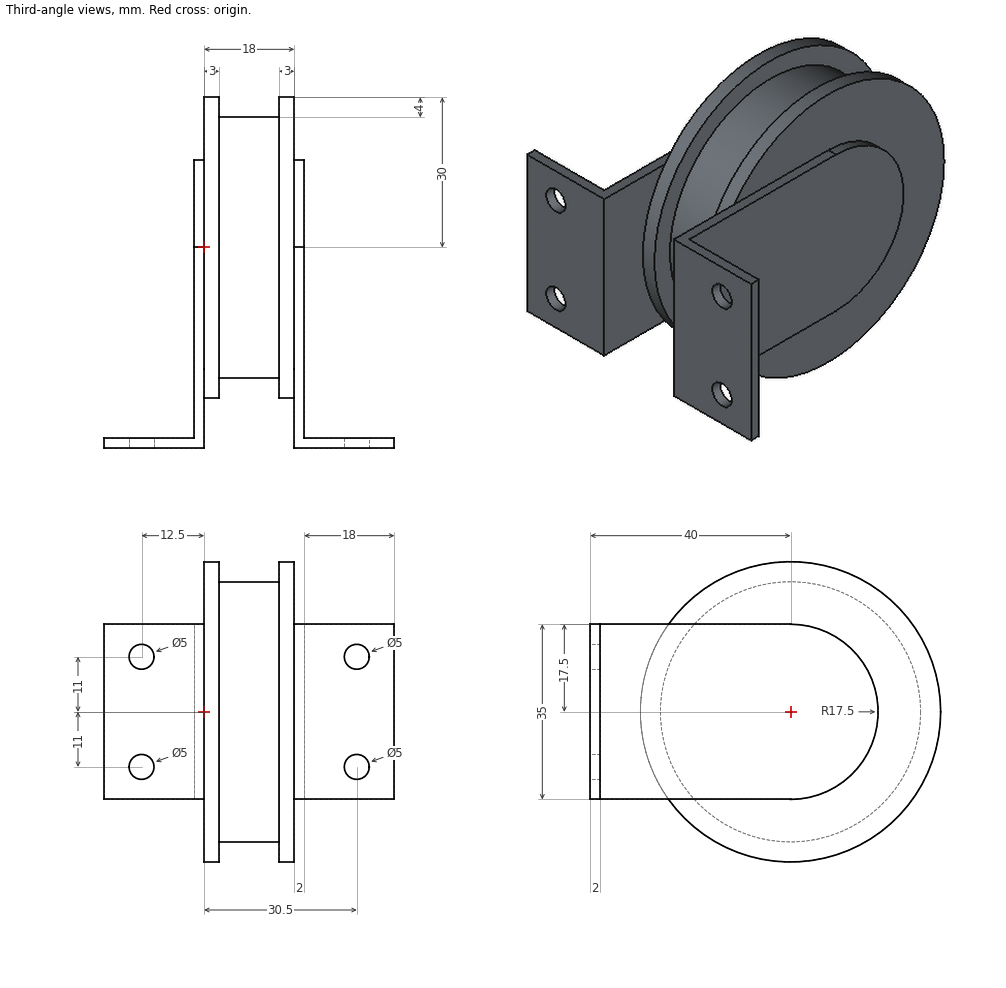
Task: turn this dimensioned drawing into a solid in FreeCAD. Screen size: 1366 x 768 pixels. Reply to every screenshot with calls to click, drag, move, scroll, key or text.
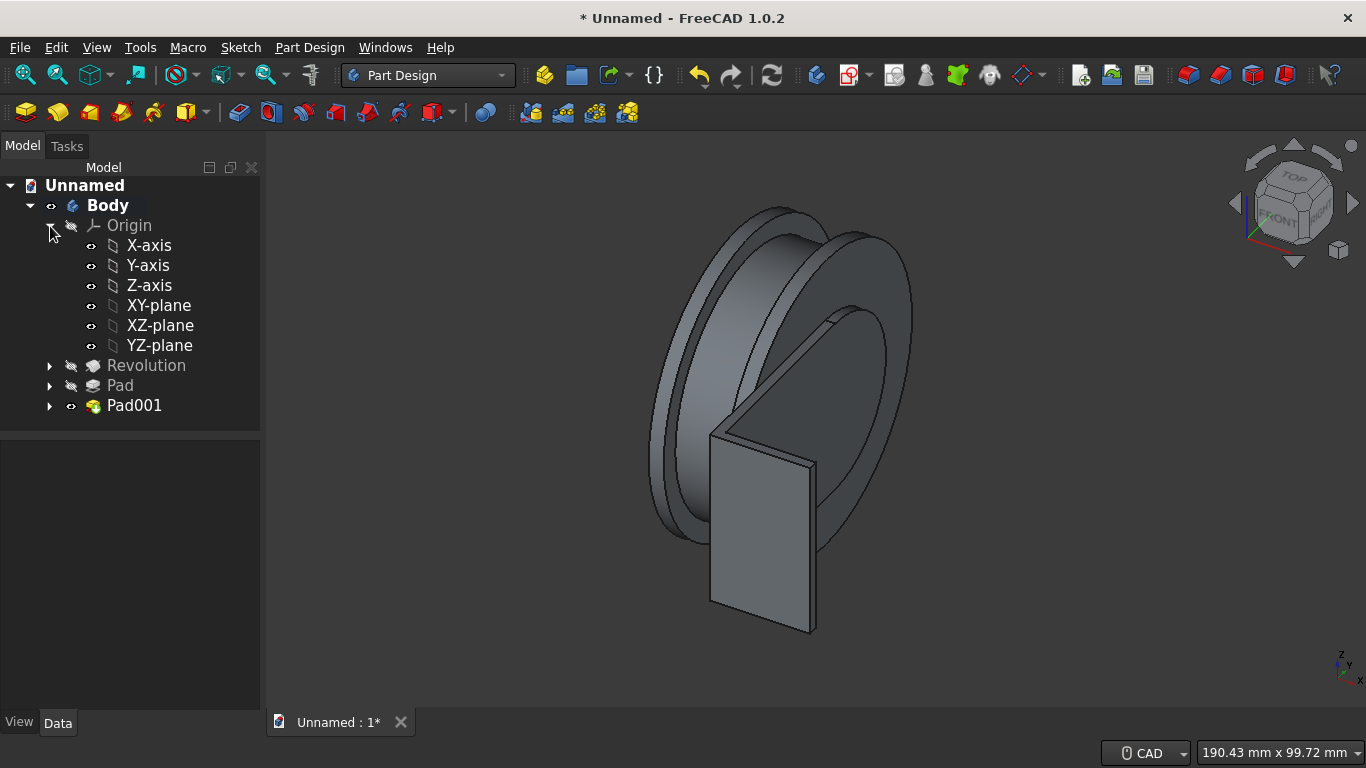
click(136, 346)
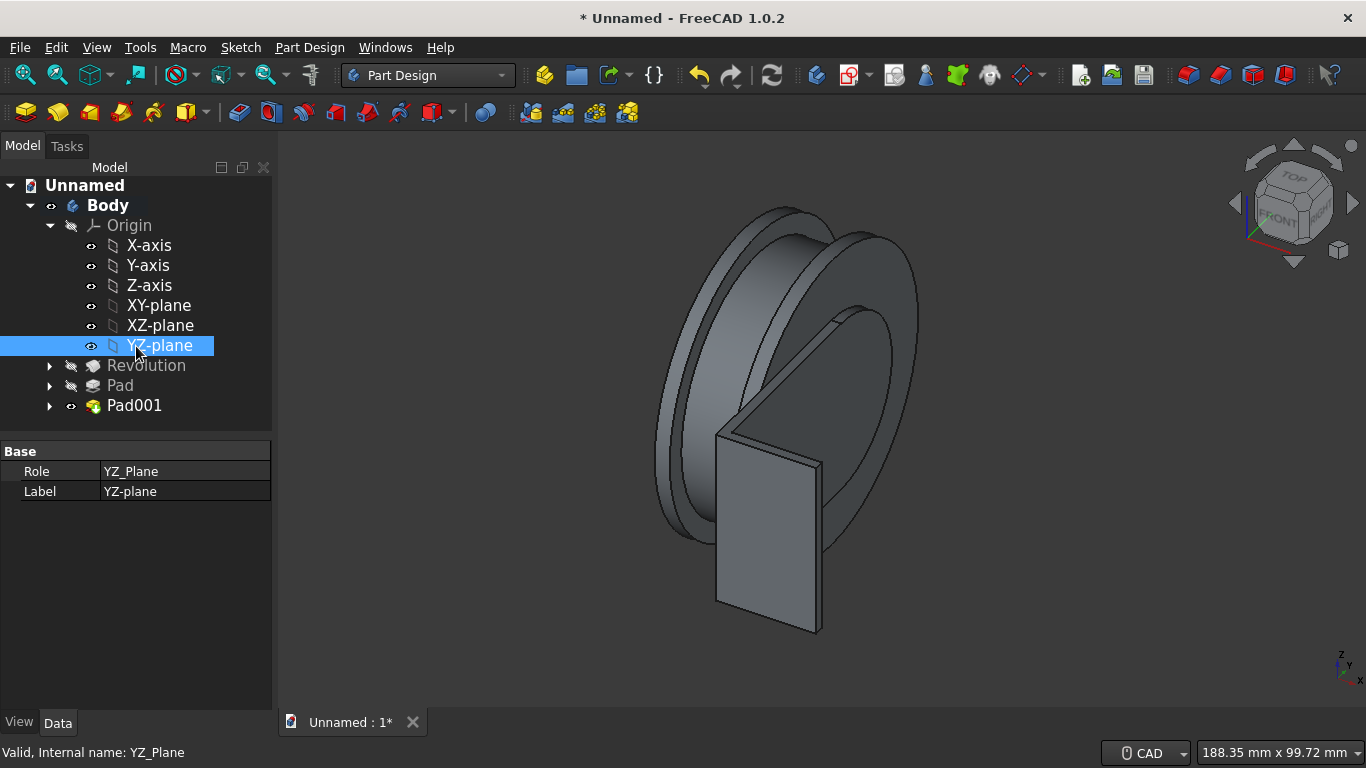
click(1022, 76)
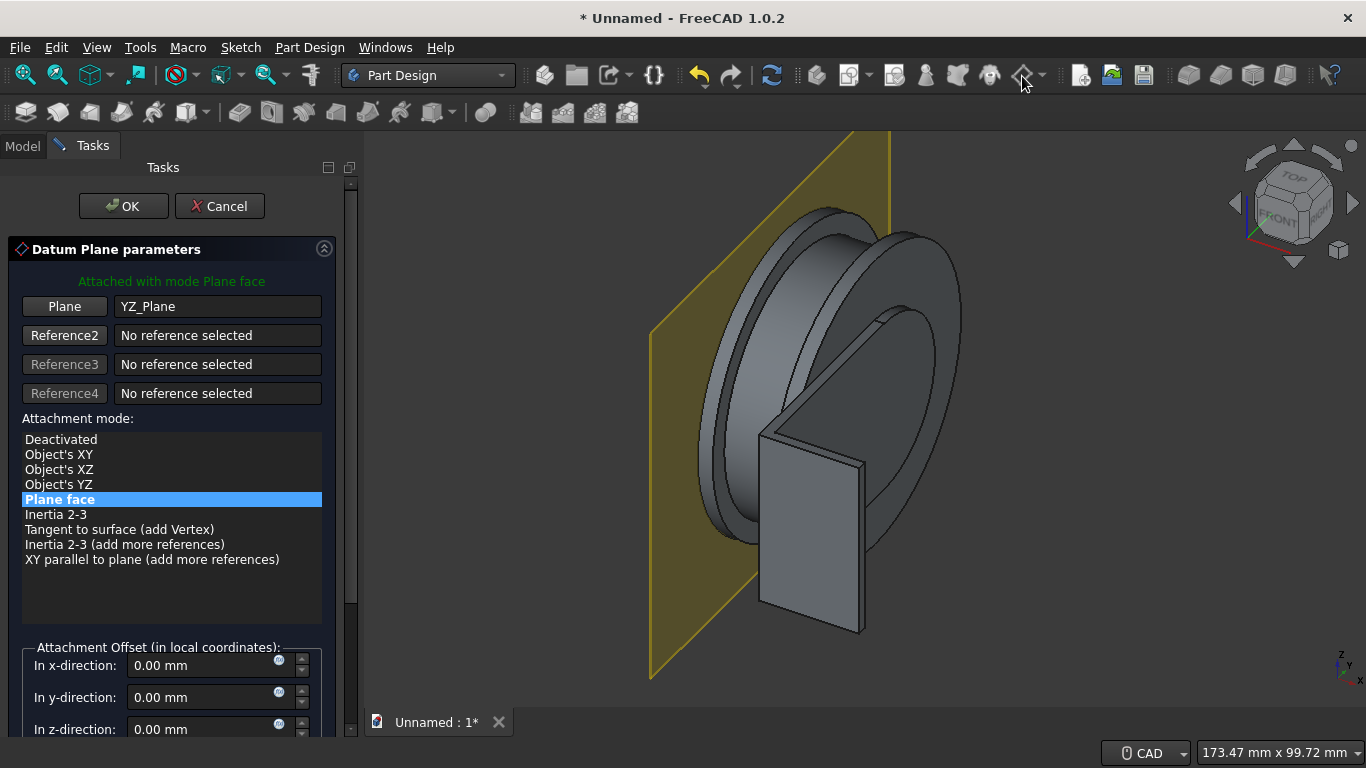
scroll(351, 456, down, 2)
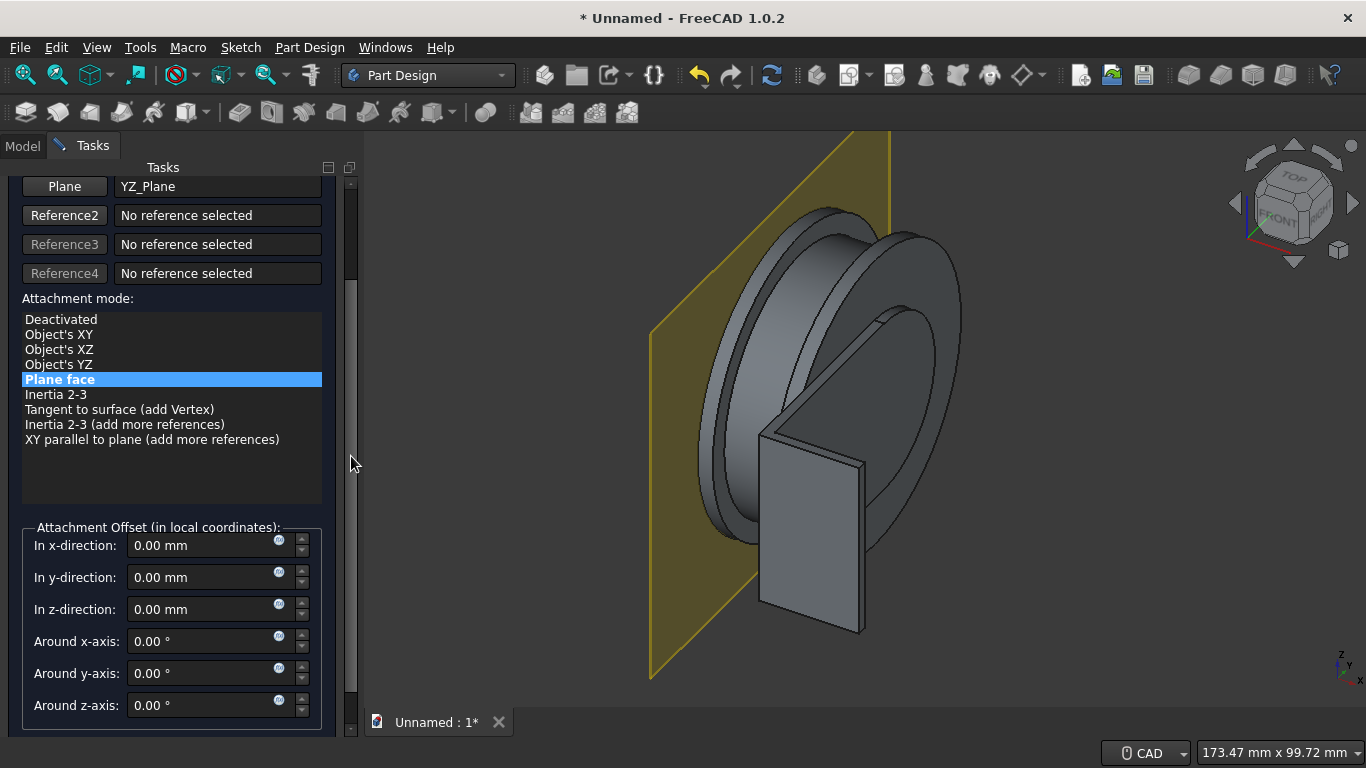
triple_click(210, 609)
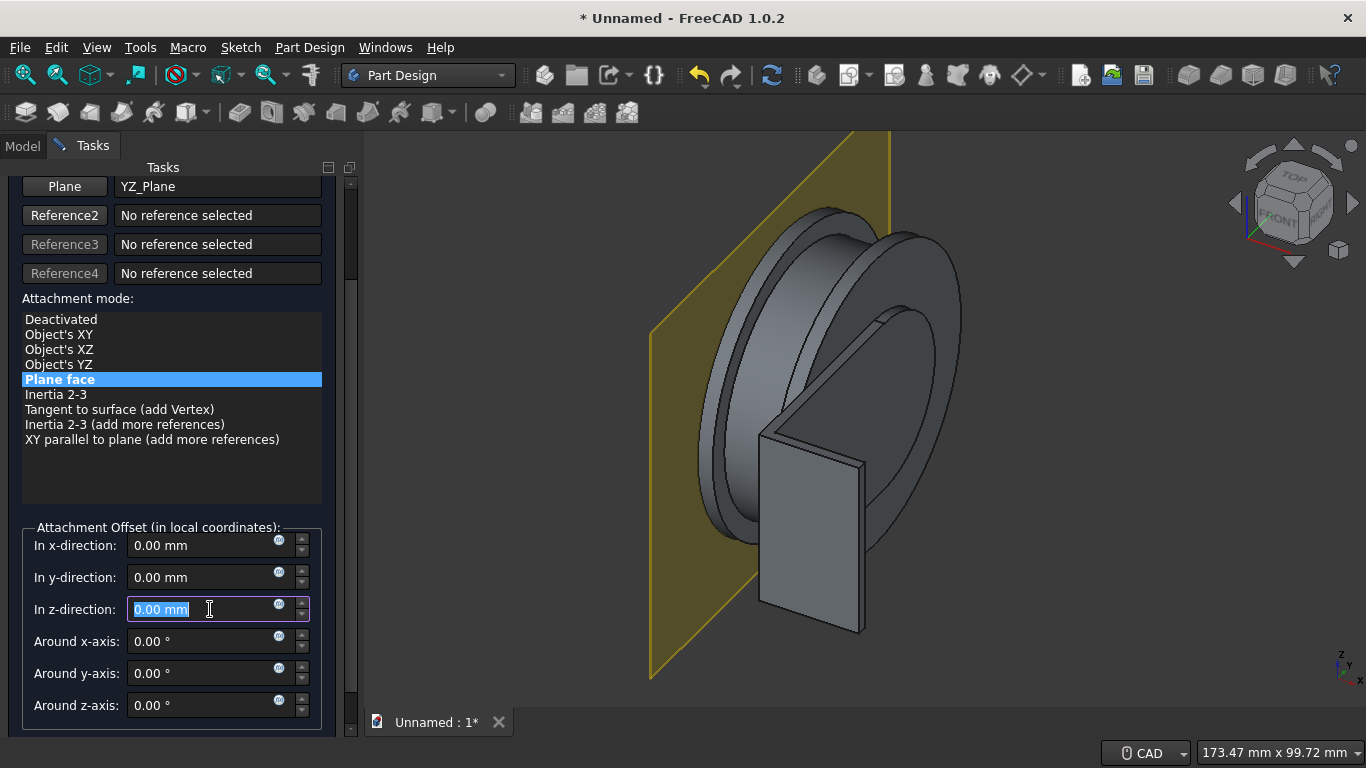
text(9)
key(Tab)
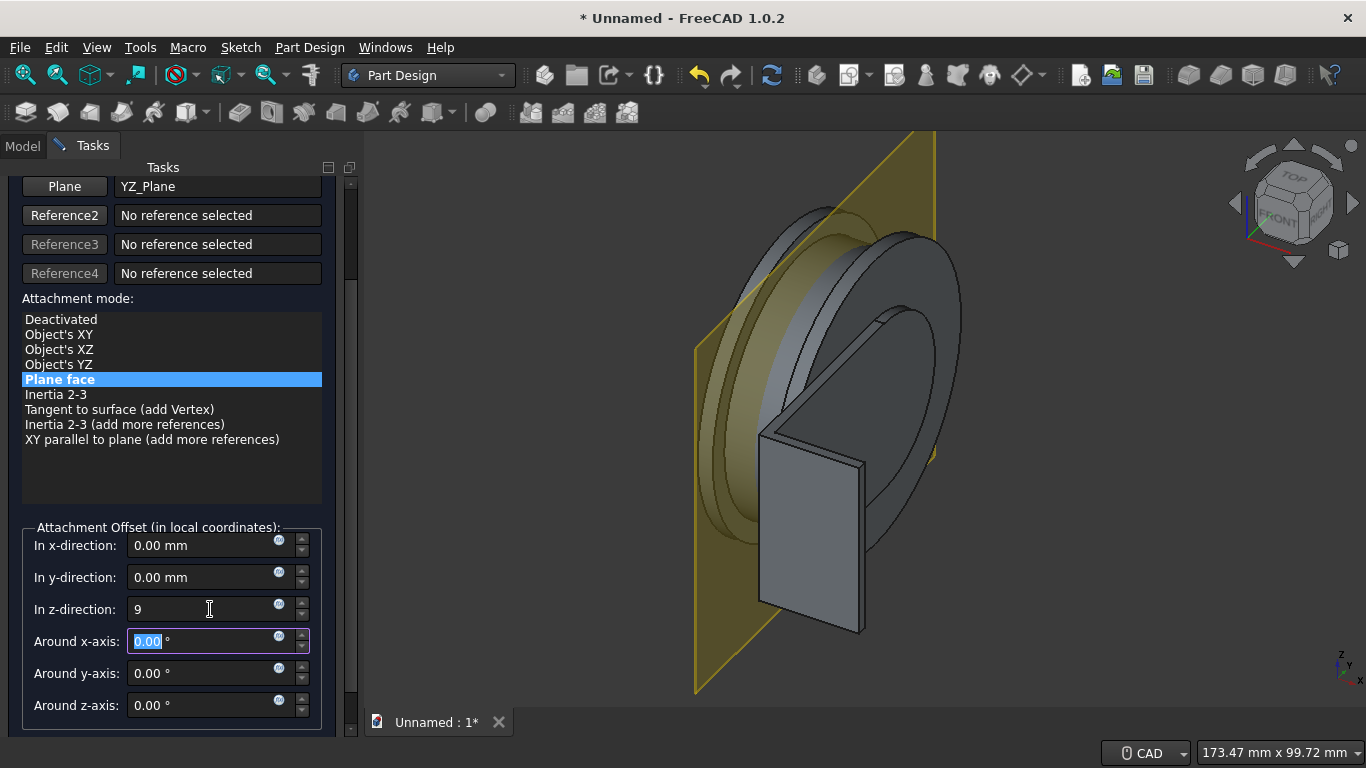
scroll(351, 456, up, 3)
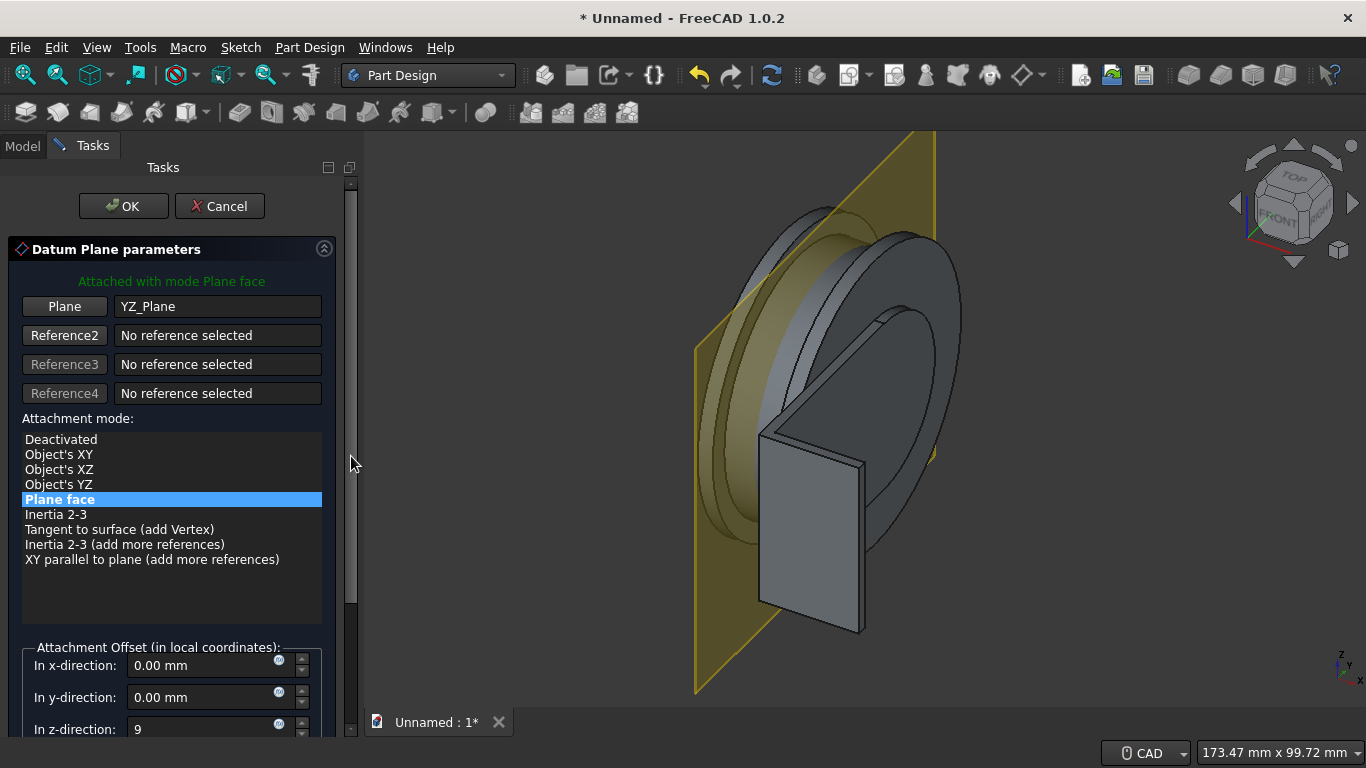
click(124, 206)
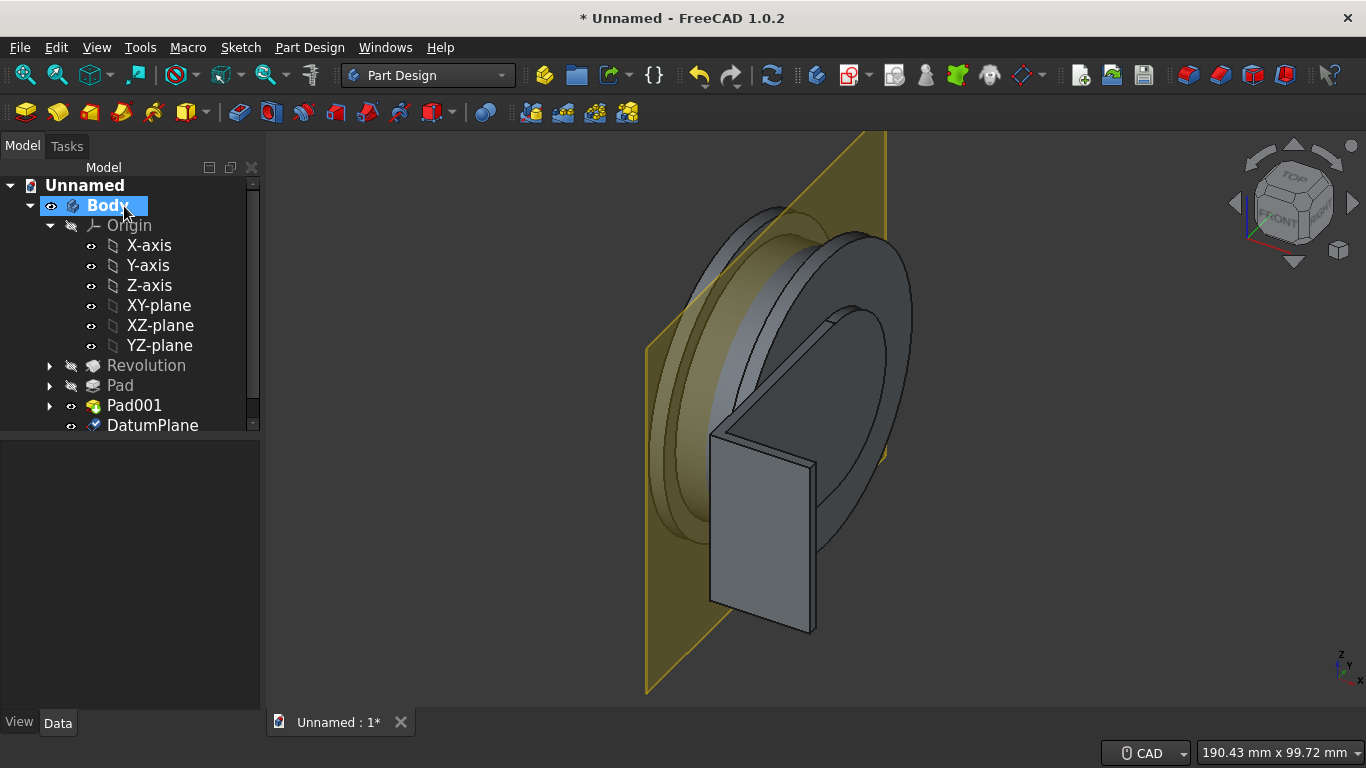
click(116, 386)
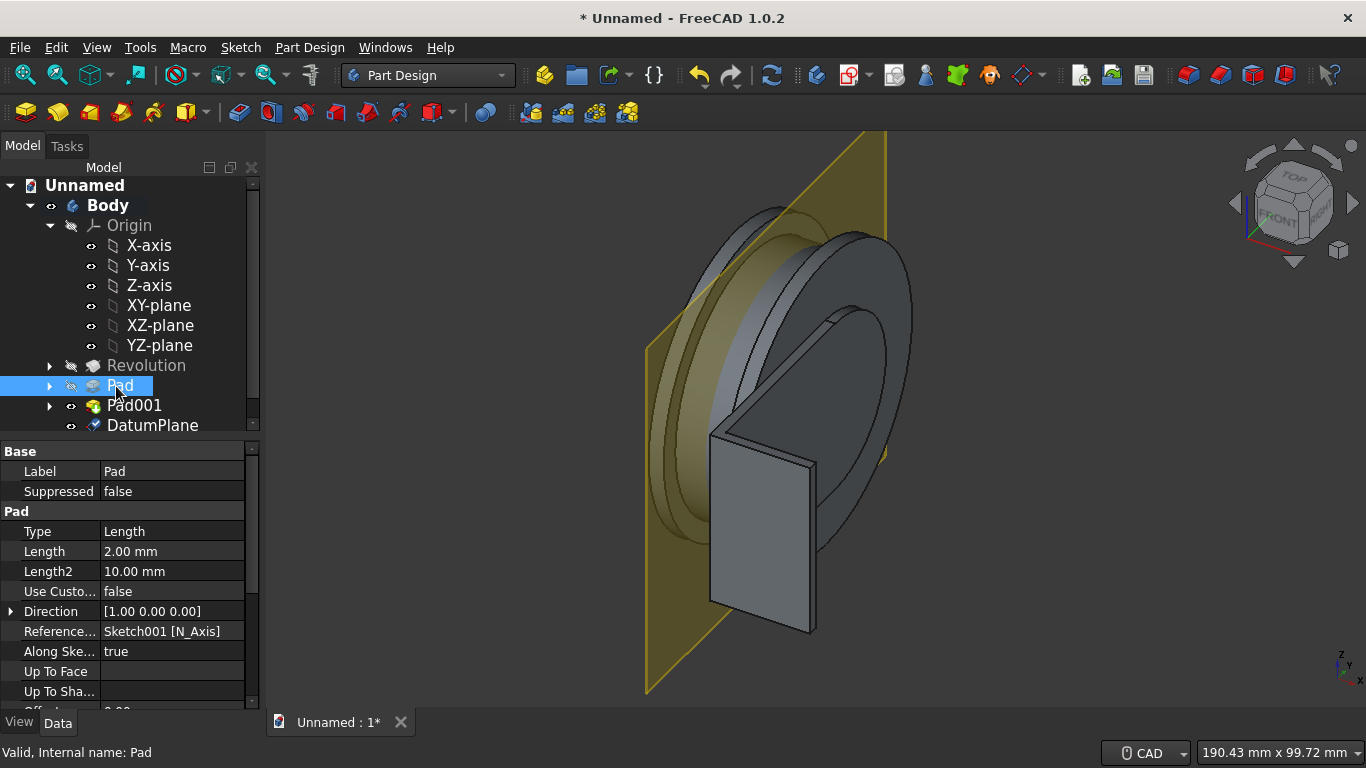
click(116, 406, ctrl)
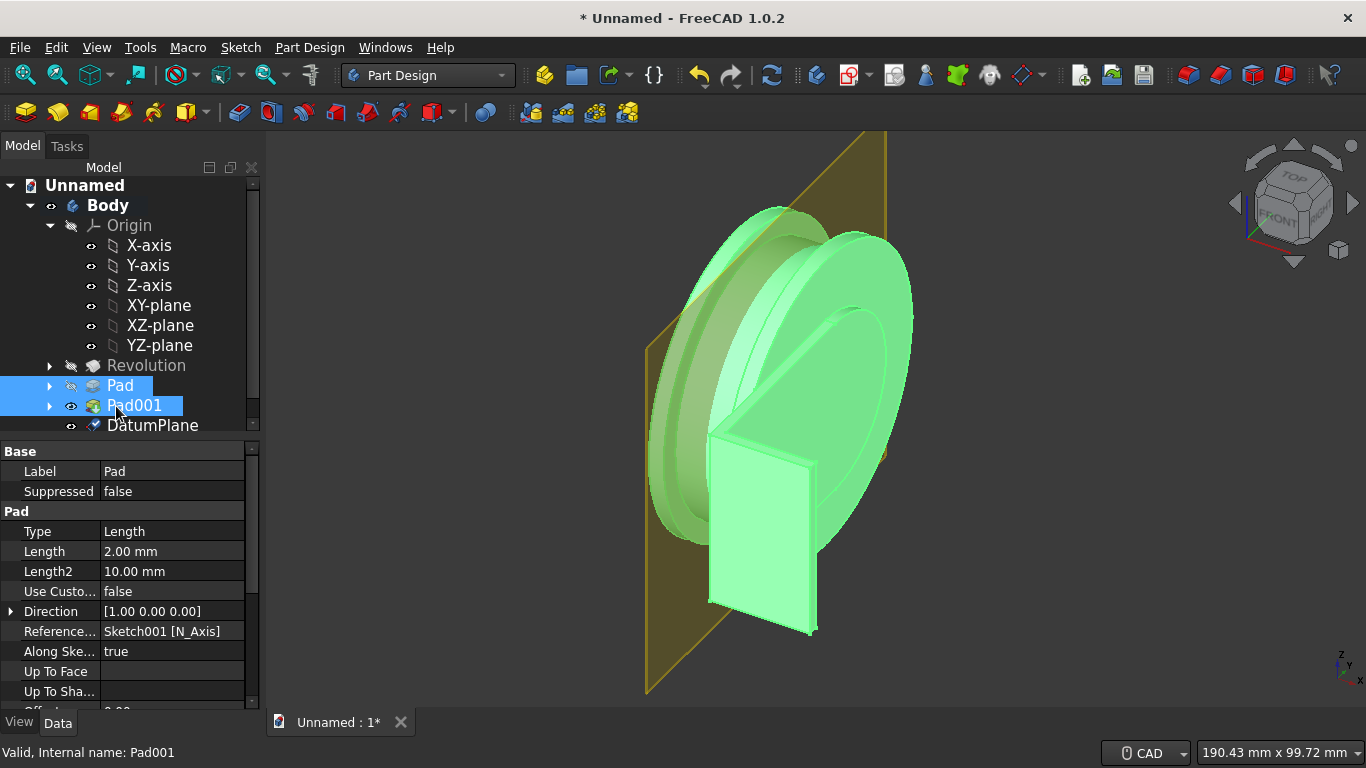
click(532, 112)